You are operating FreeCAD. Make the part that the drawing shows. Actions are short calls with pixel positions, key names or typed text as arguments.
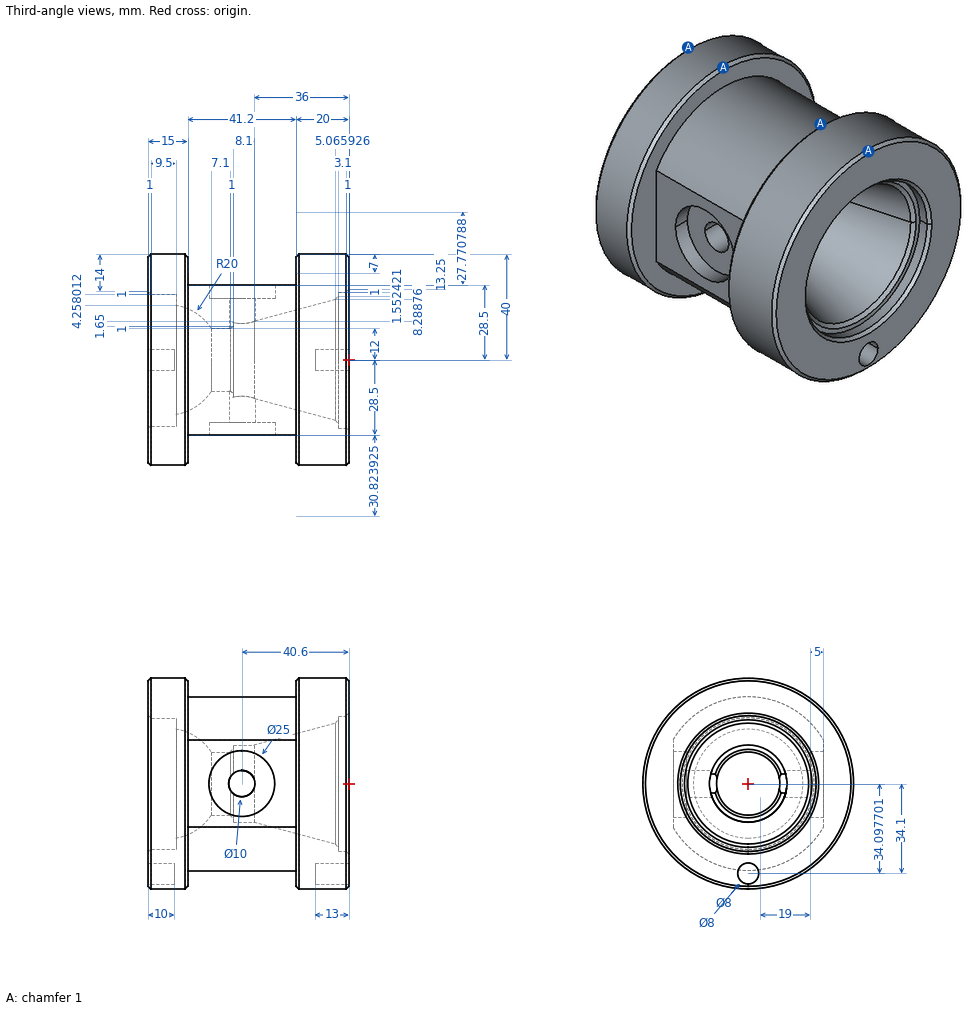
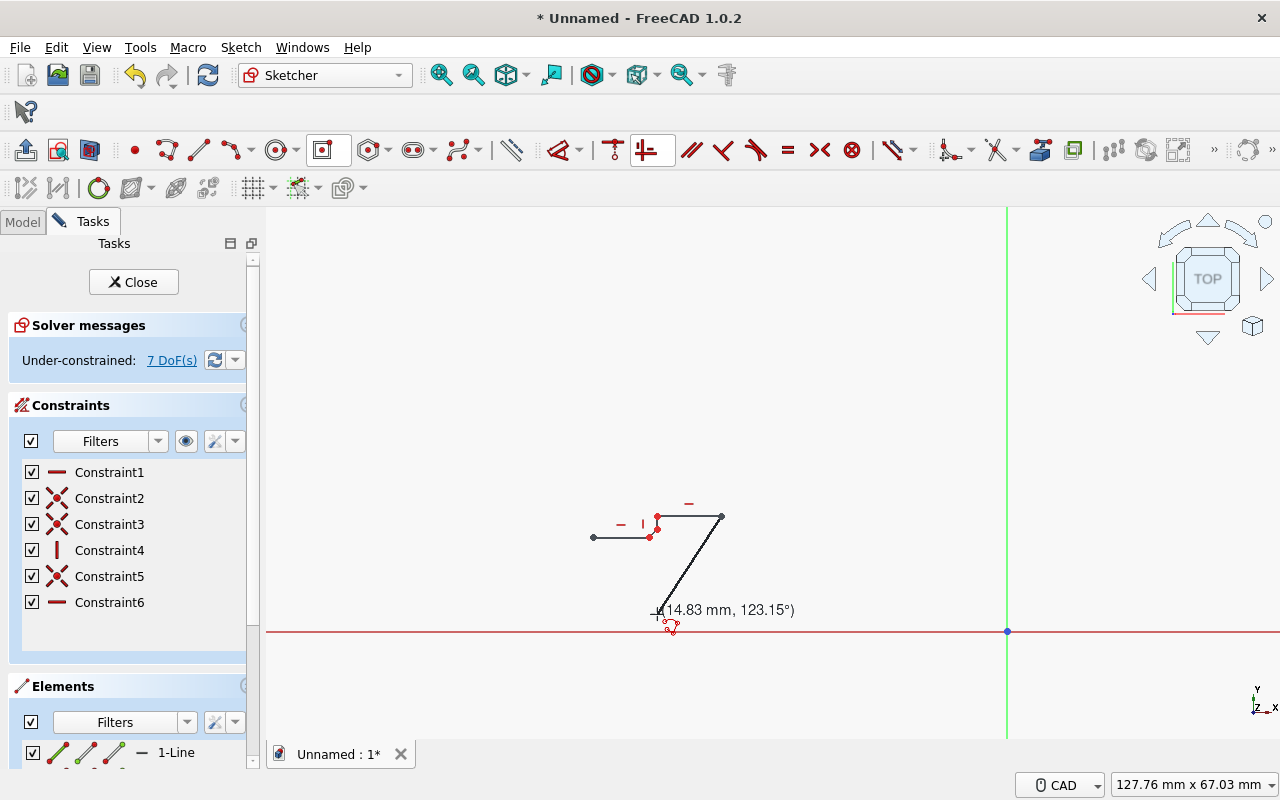
click(967, 450)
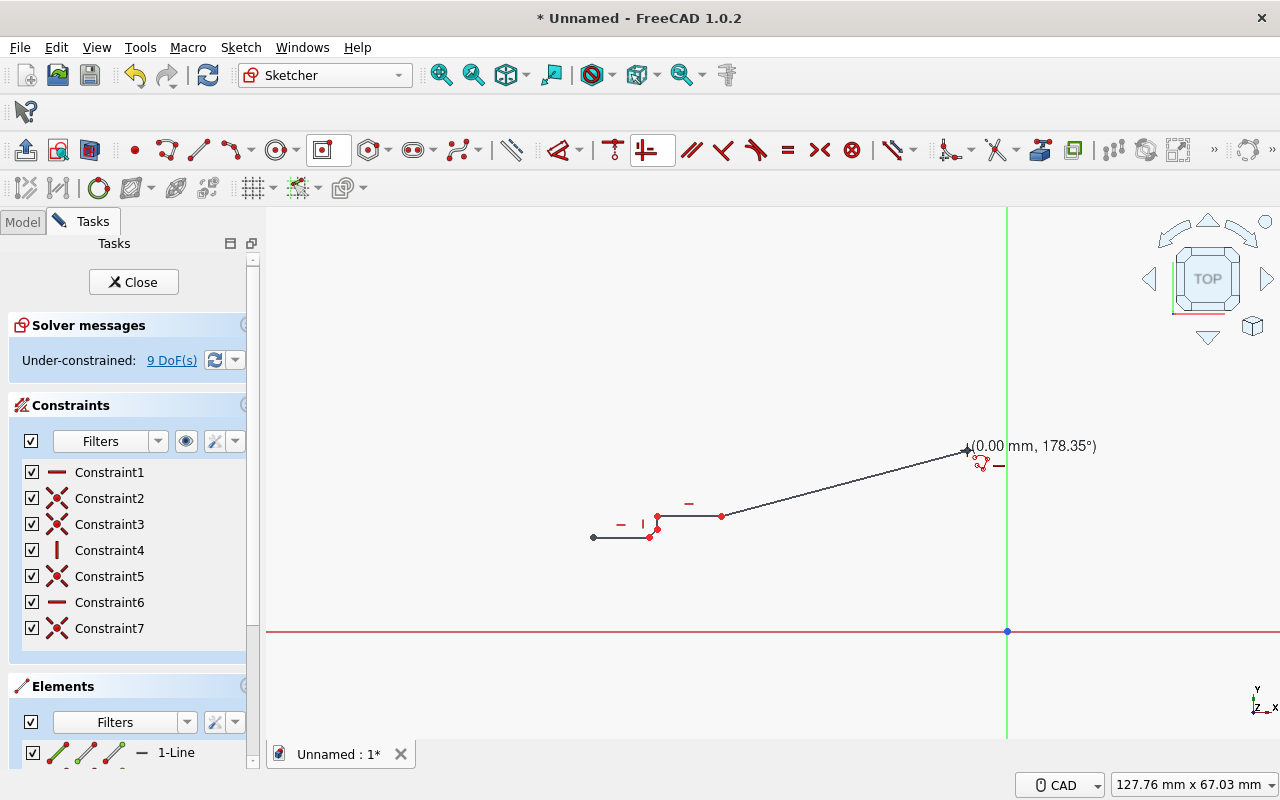
scroll(975, 440, up, 2)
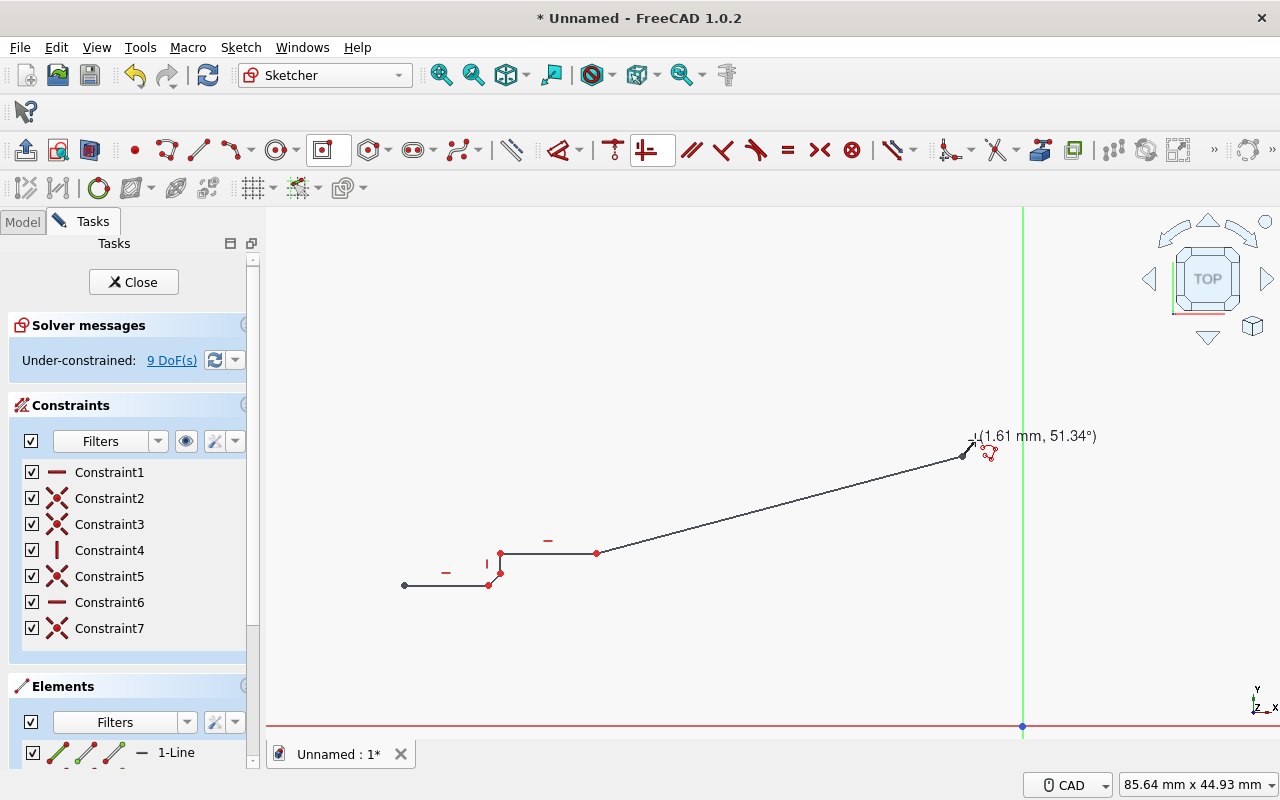
click(974, 440)
click(974, 421)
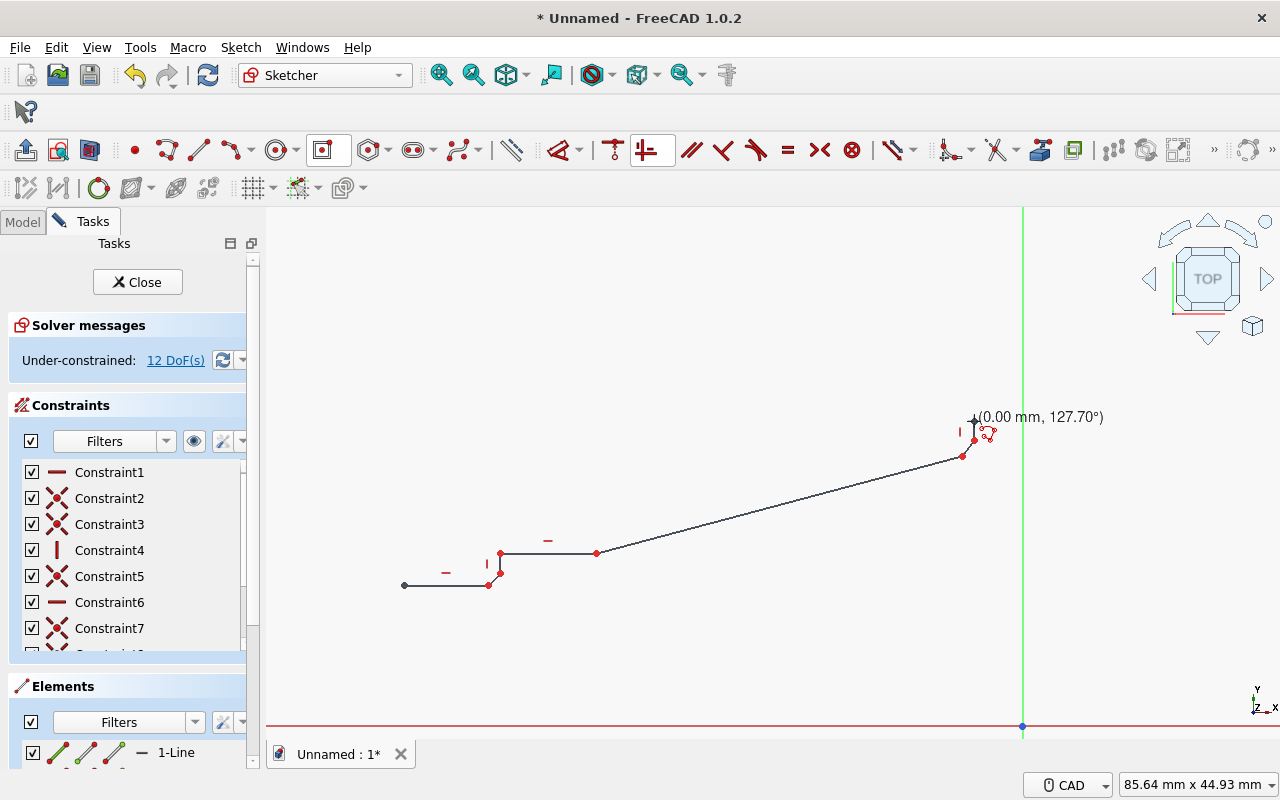
scroll(1011, 421, up, 2)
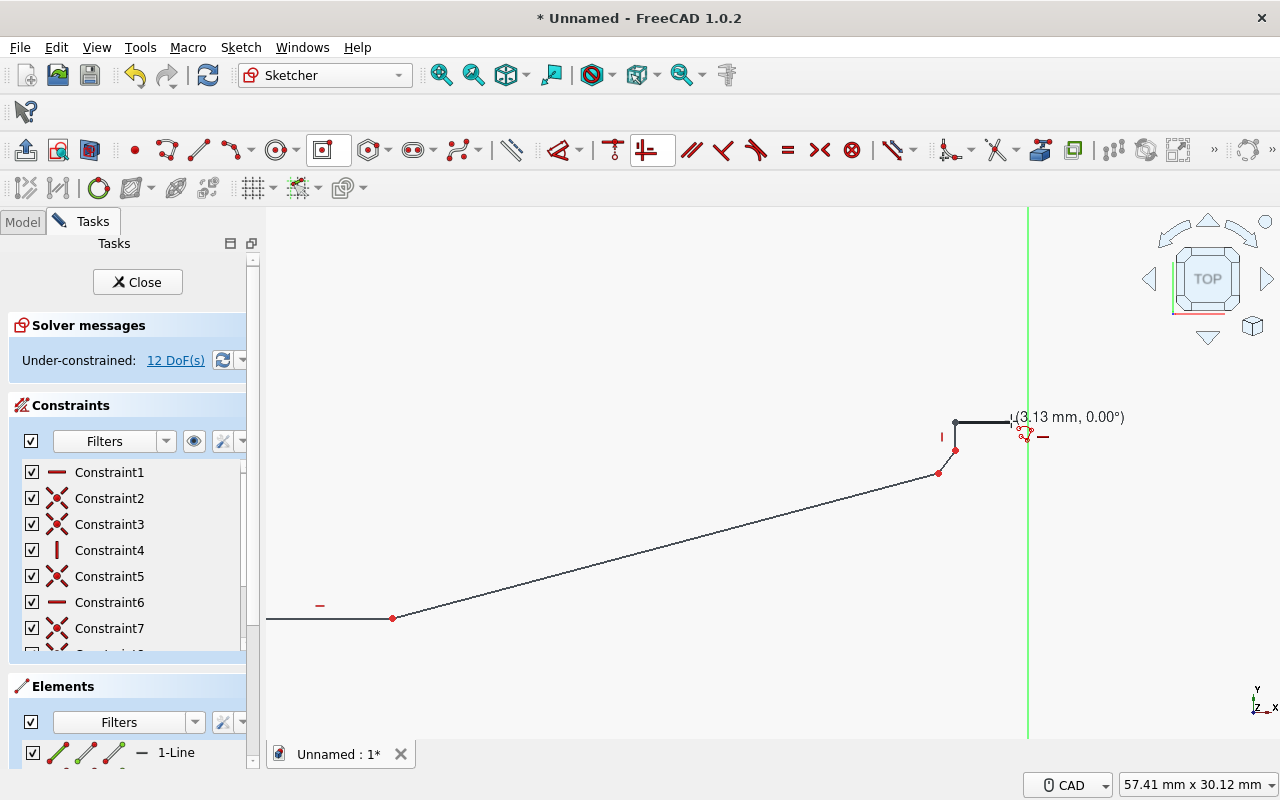
click(1010, 421)
click(1028, 404)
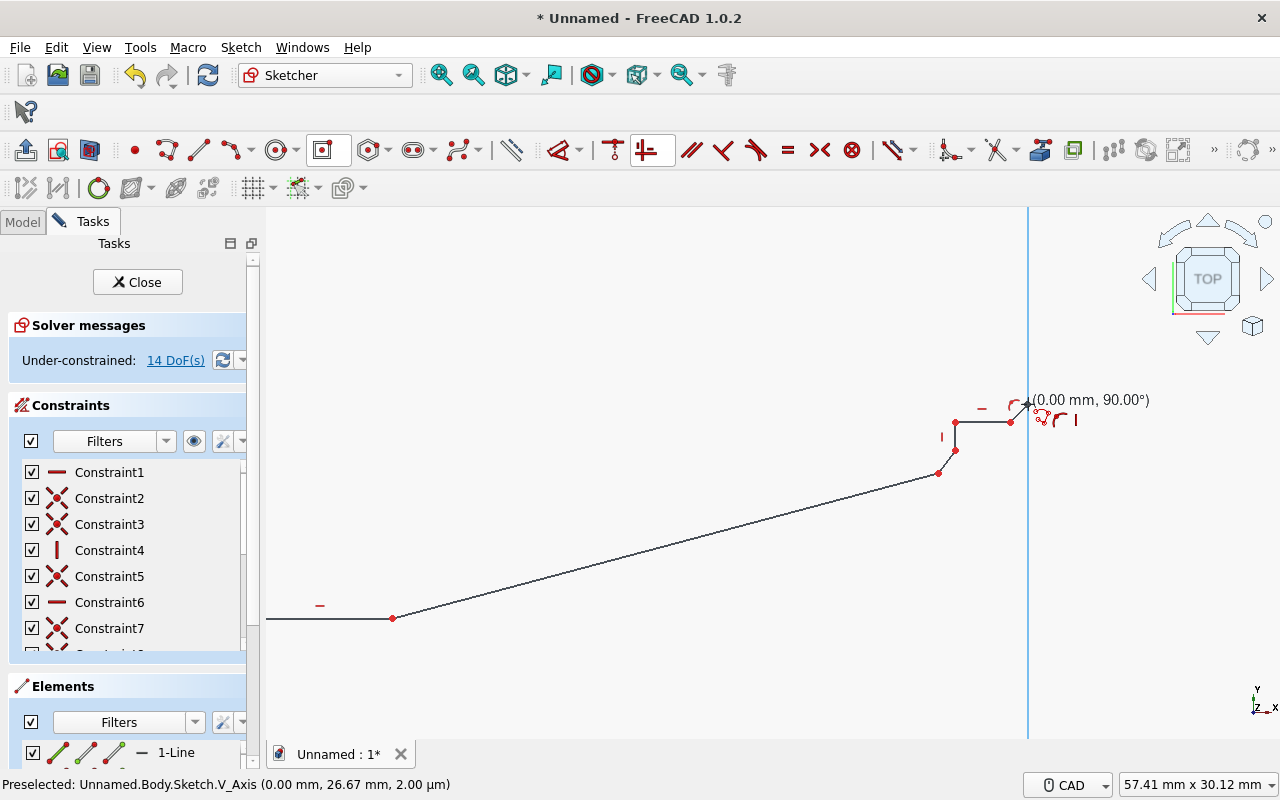
scroll(990, 432, down, 4)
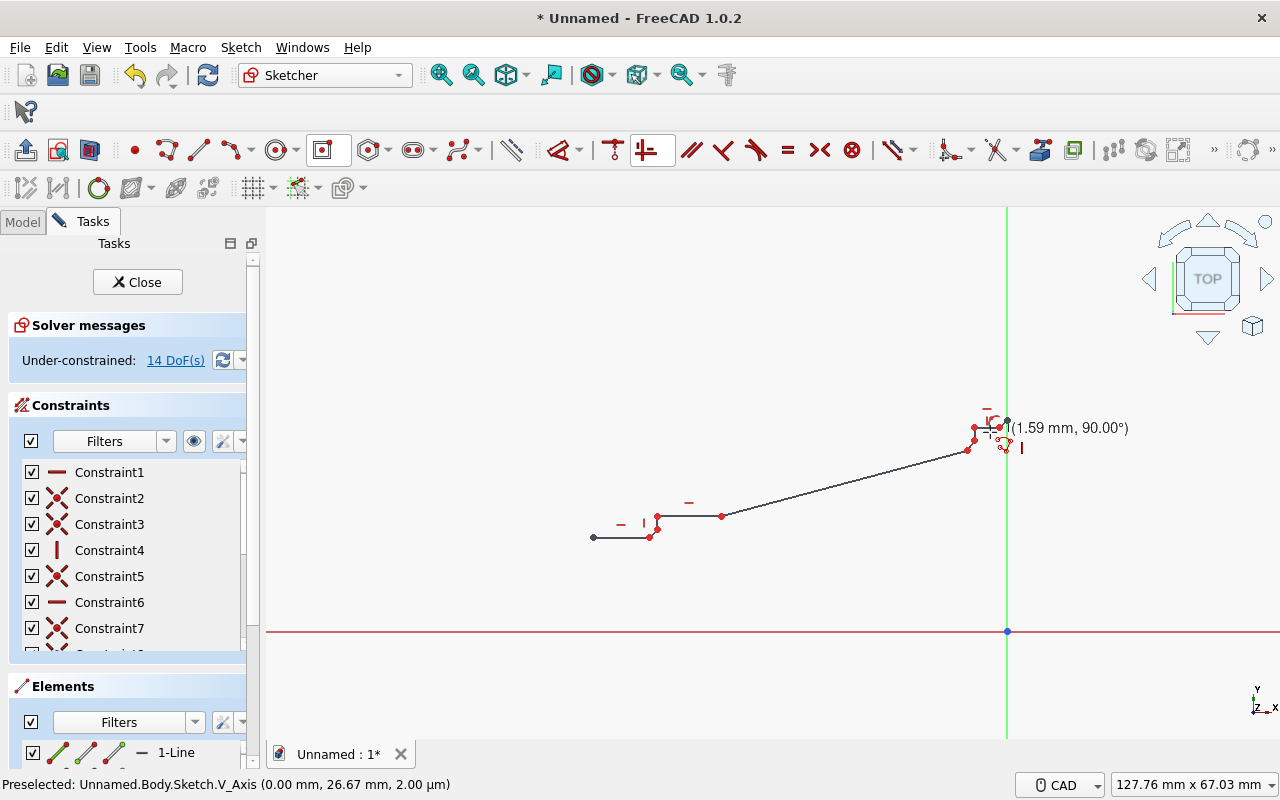
click(998, 314)
click(849, 314)
click(849, 370)
click(522, 370)
click(522, 314)
click(403, 314)
click(403, 425)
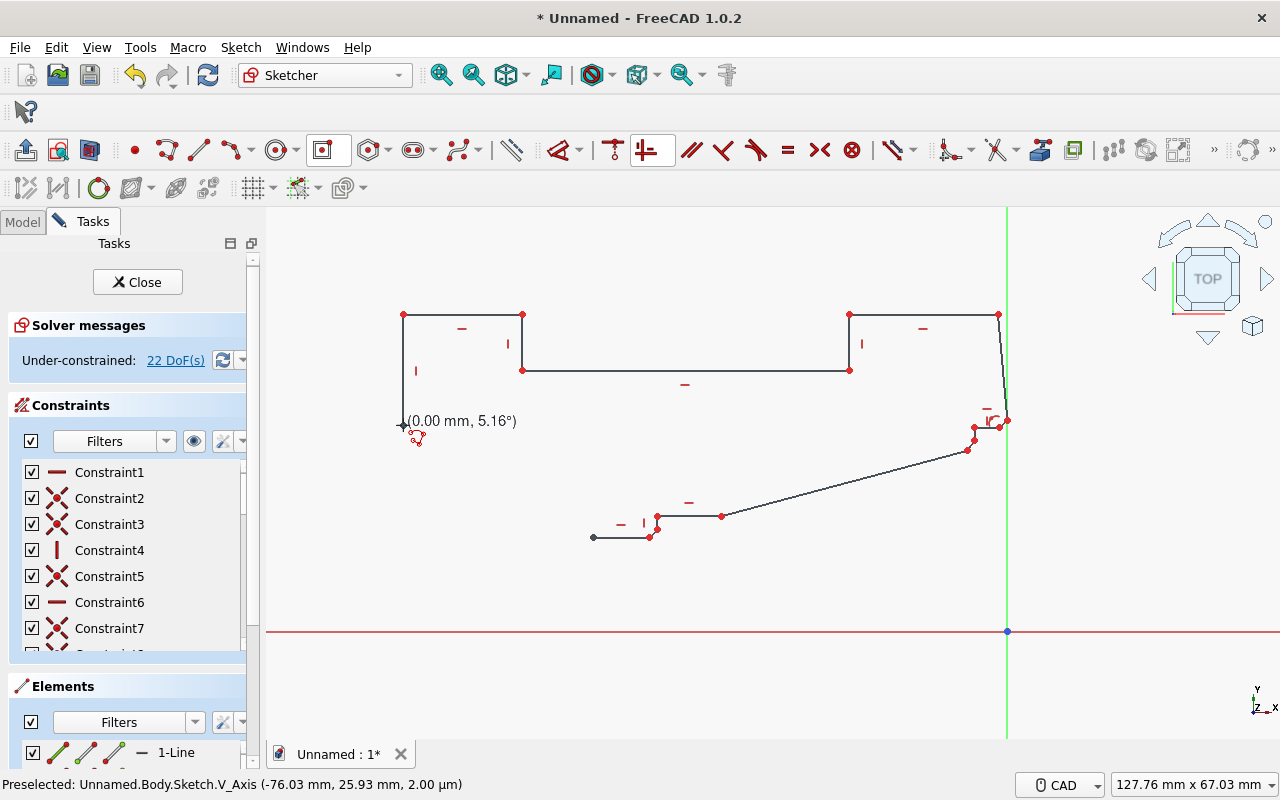
scroll(411, 433, up, 2)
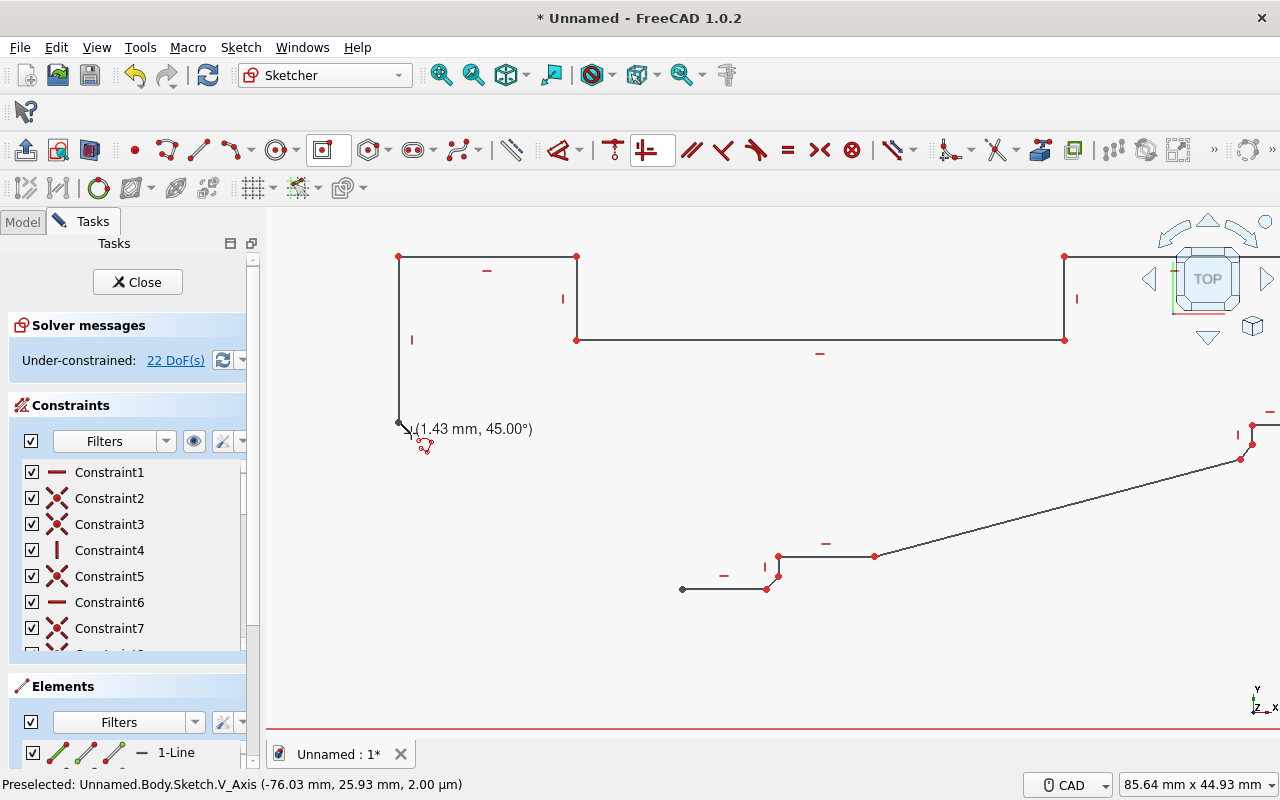
click(410, 433)
click(523, 433)
click(523, 484)
right_click(523, 484)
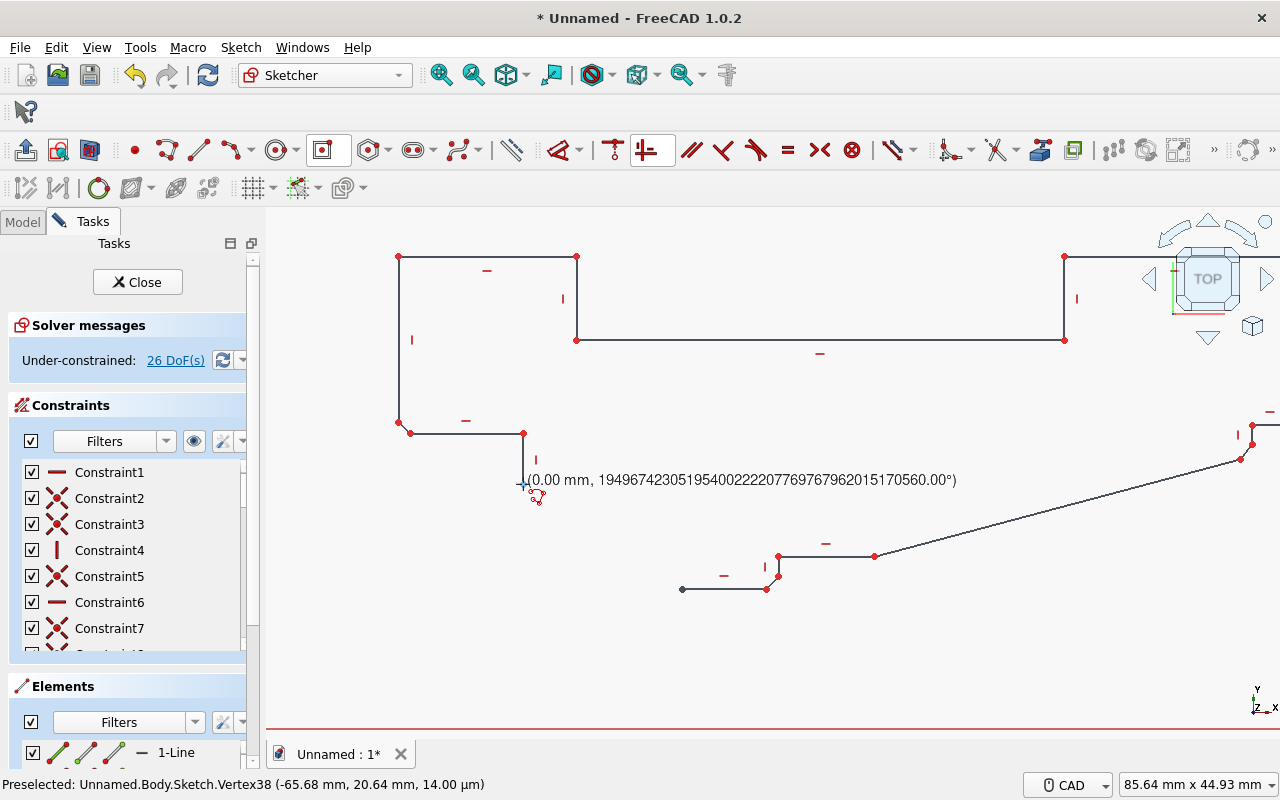
click(232, 150)